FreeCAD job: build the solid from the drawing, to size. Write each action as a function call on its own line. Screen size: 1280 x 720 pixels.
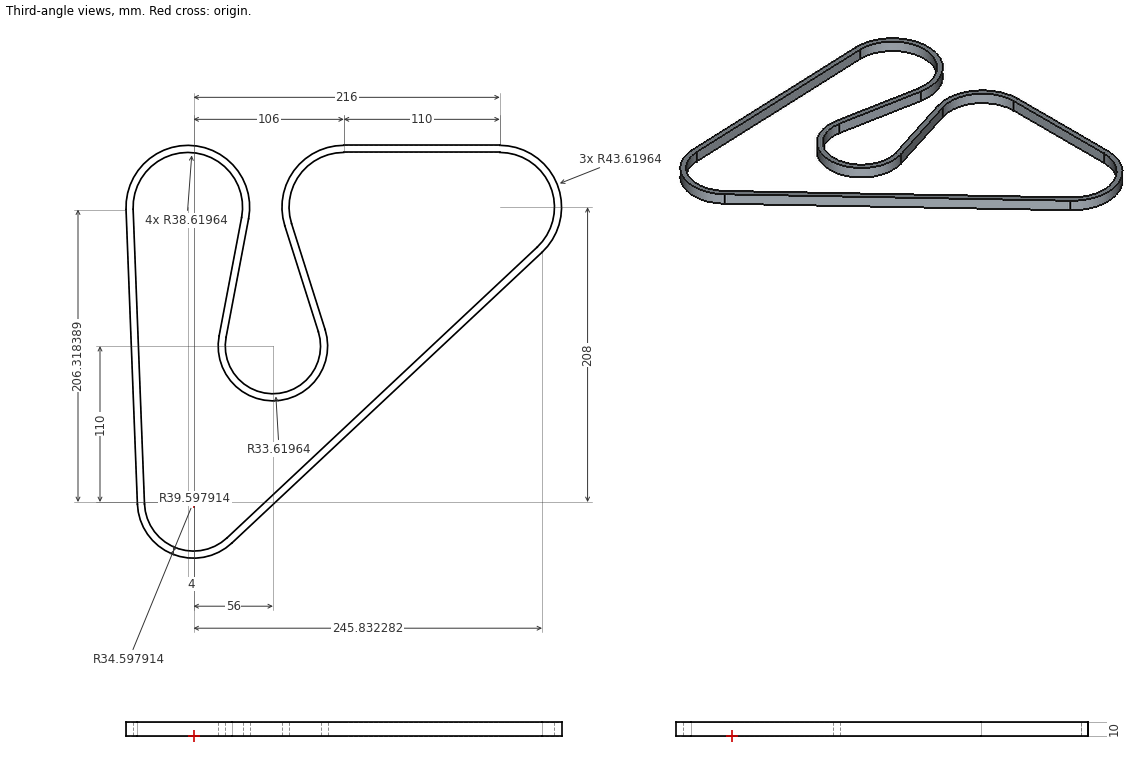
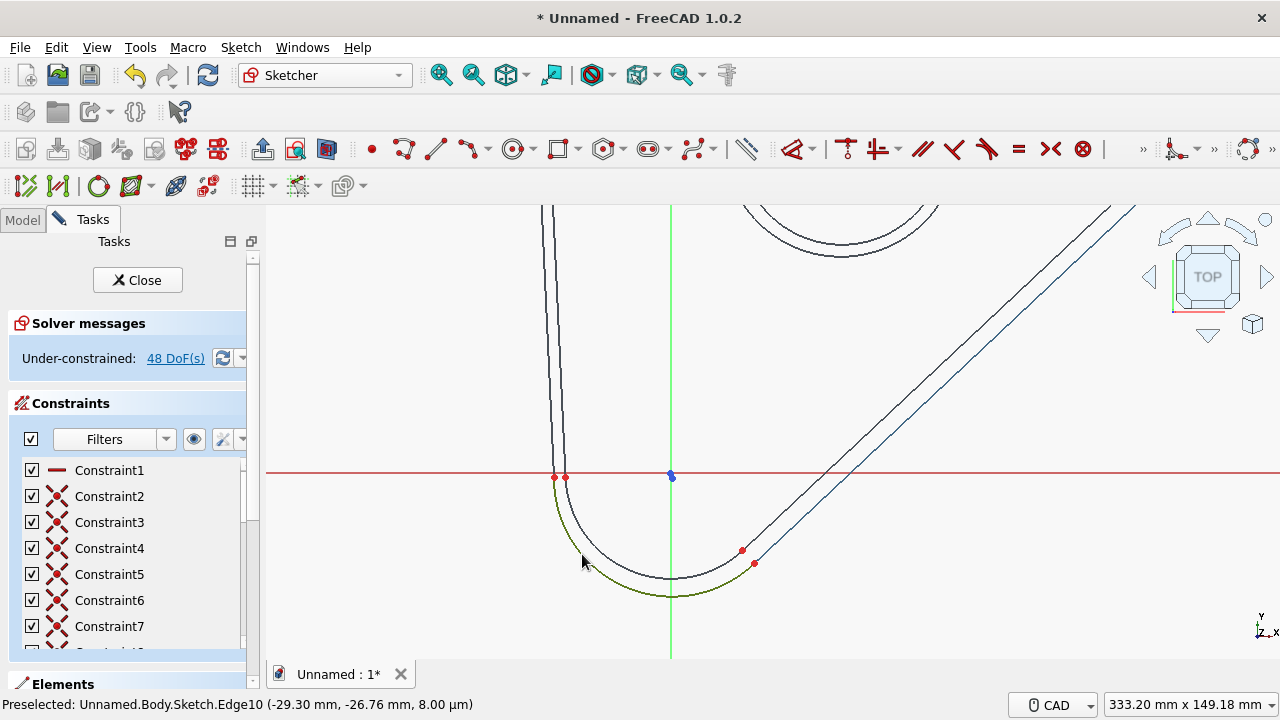
click(988, 150)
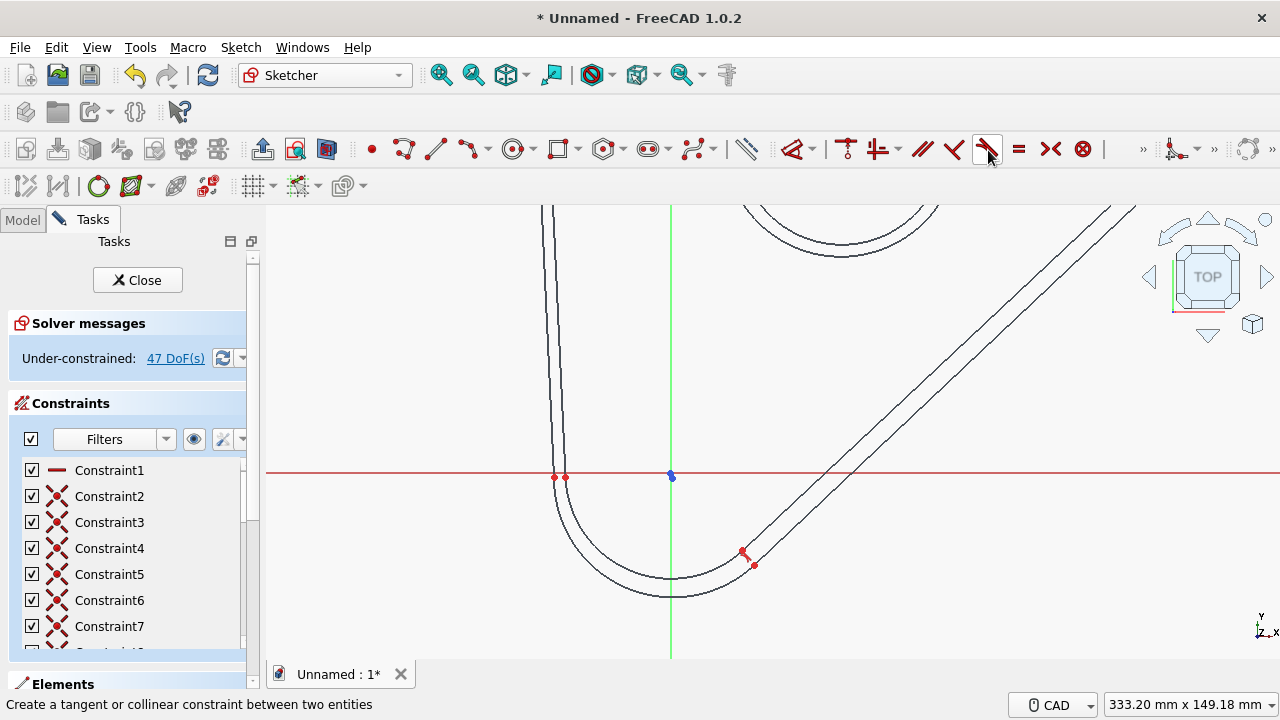
scroll(582, 555, down, 6)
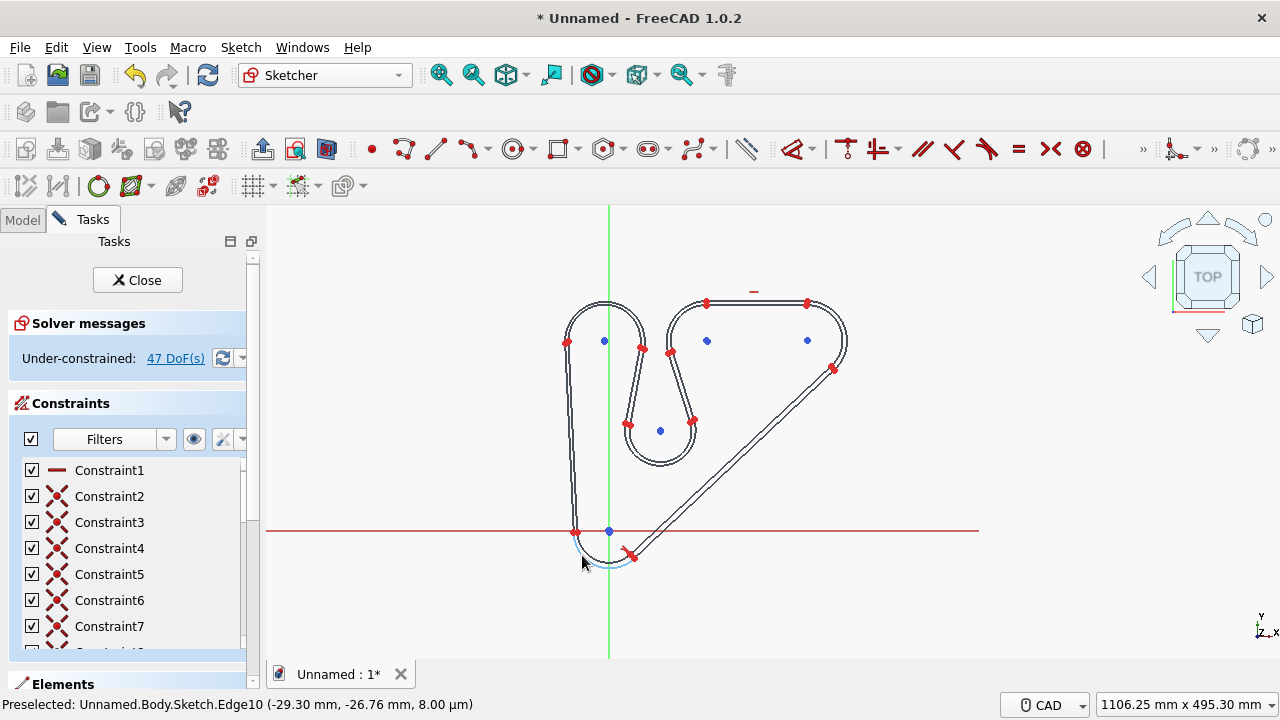
scroll(675, 374, up, 6)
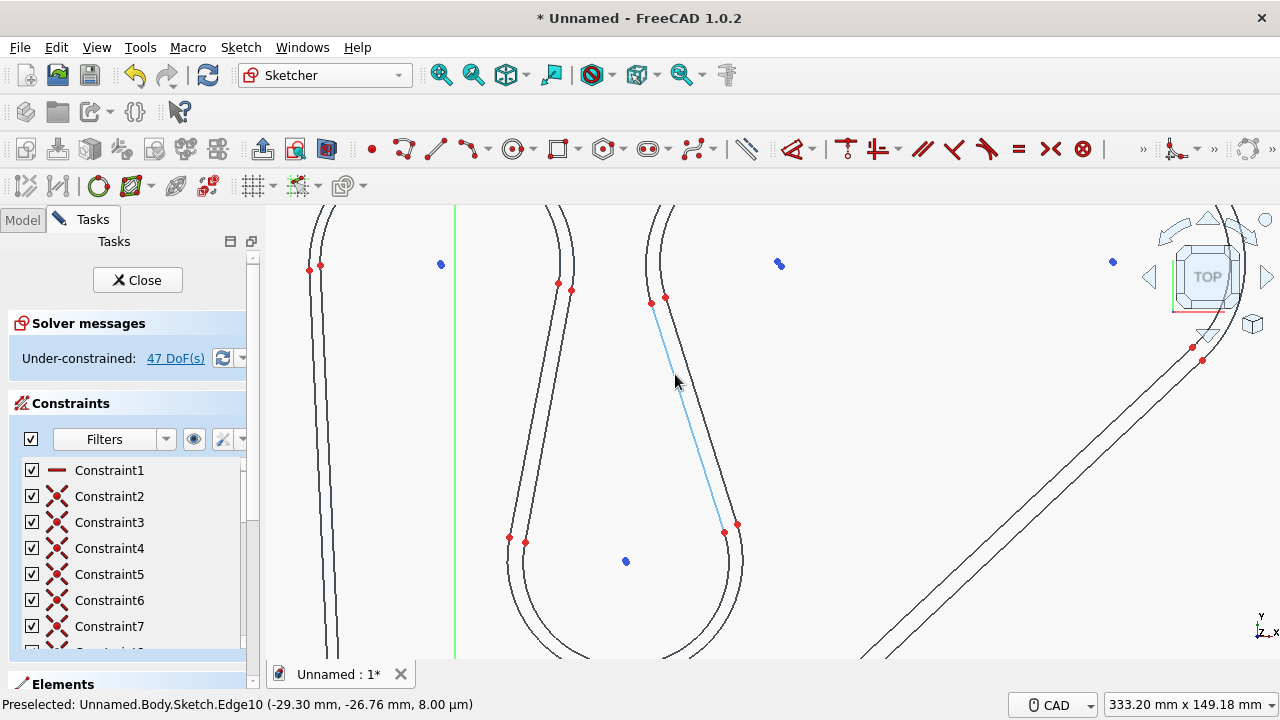
click(673, 372)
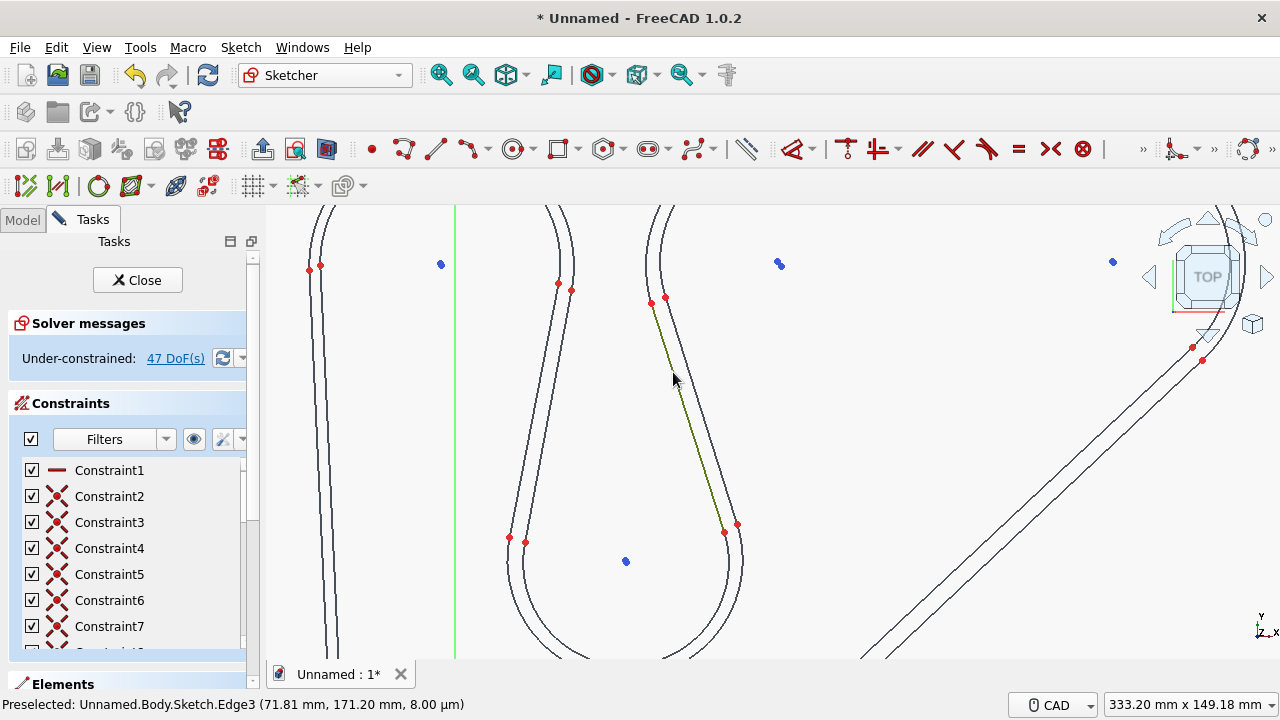
click(646, 255)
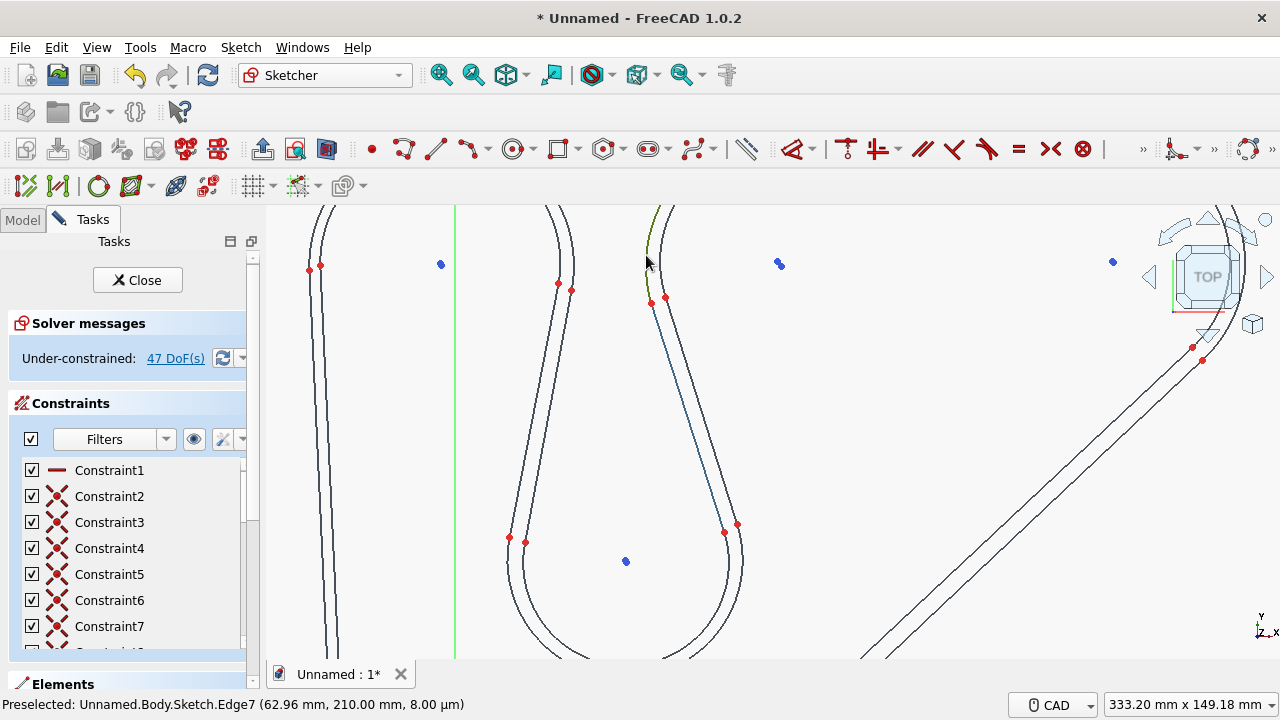
click(988, 150)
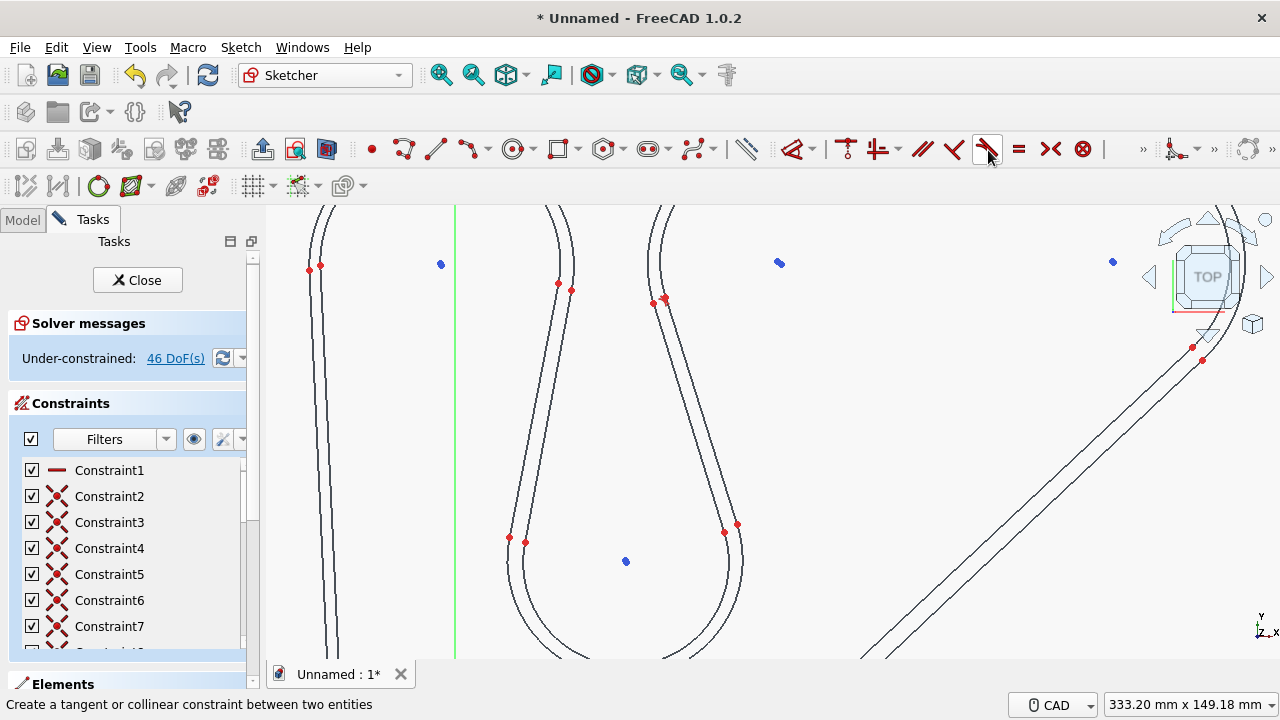
click(675, 372)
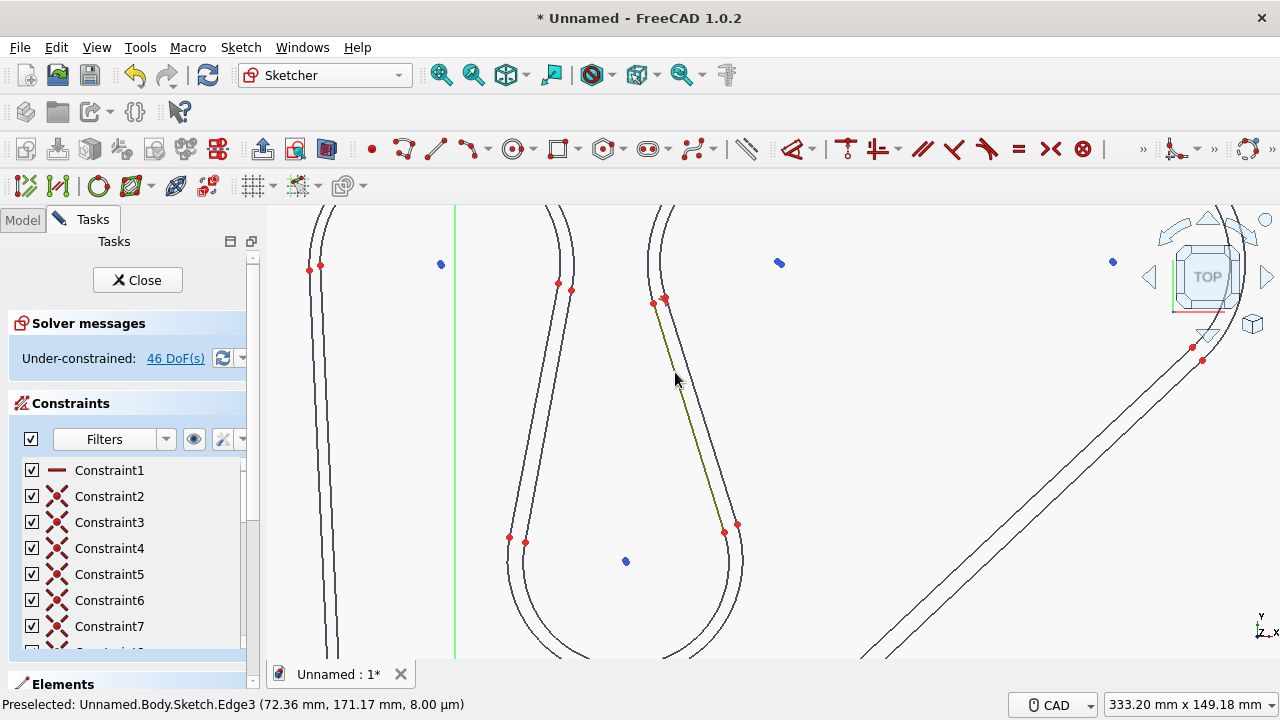
click(537, 615)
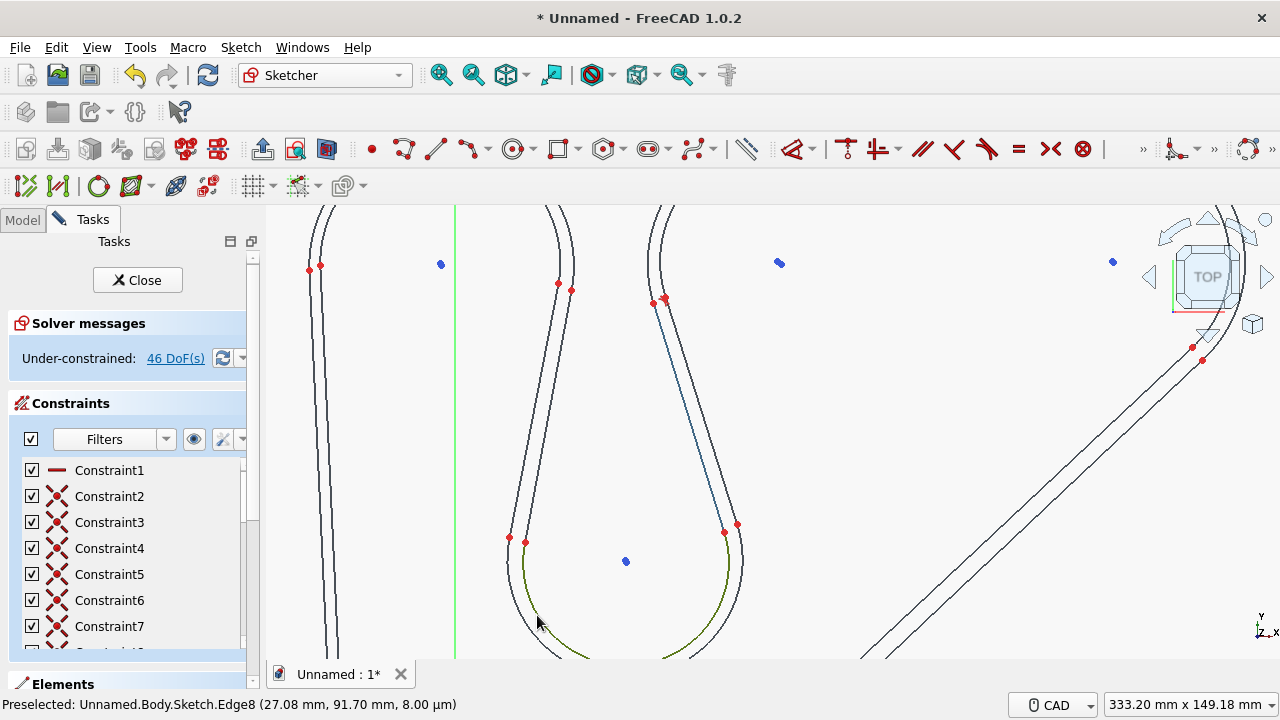
key(t)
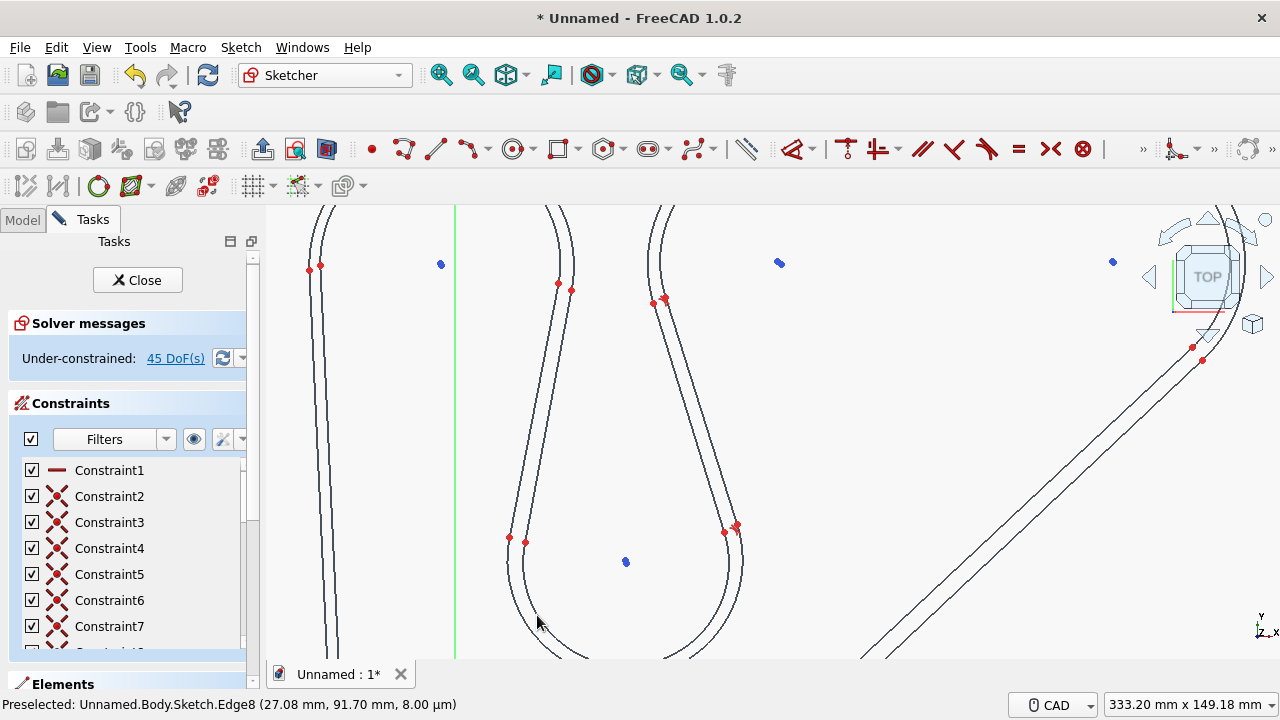
click(539, 467)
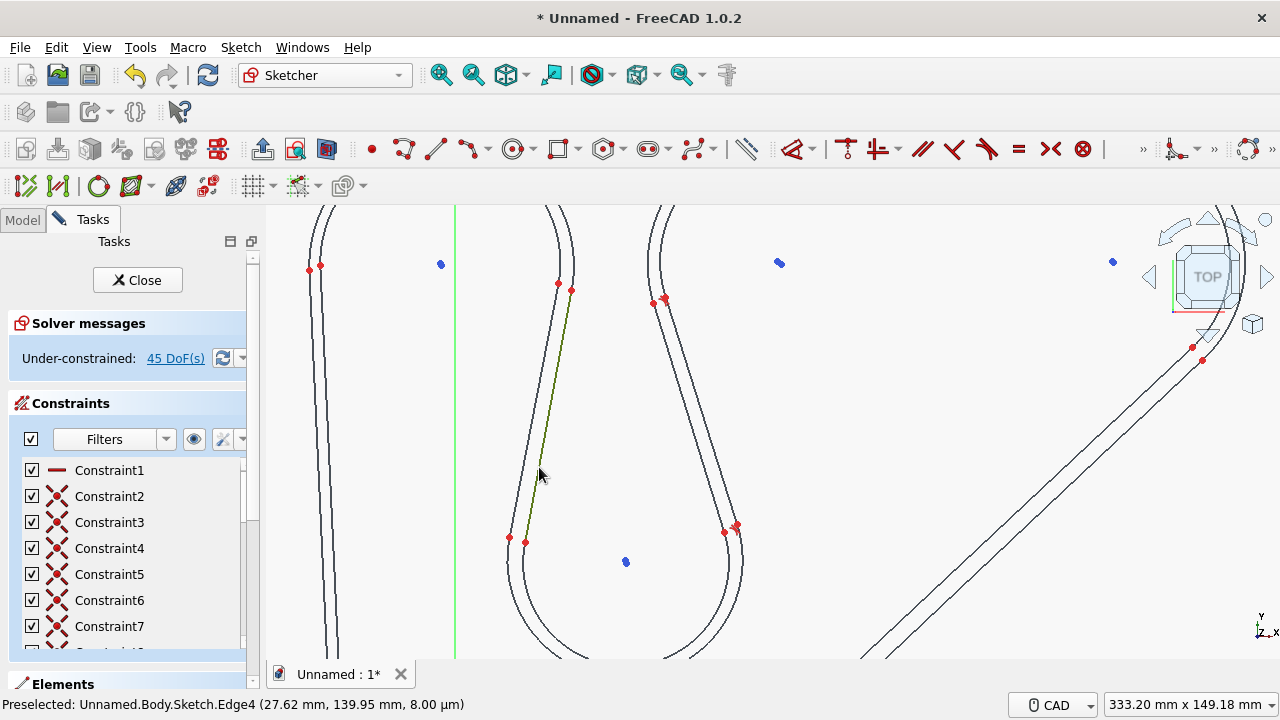
click(537, 615)